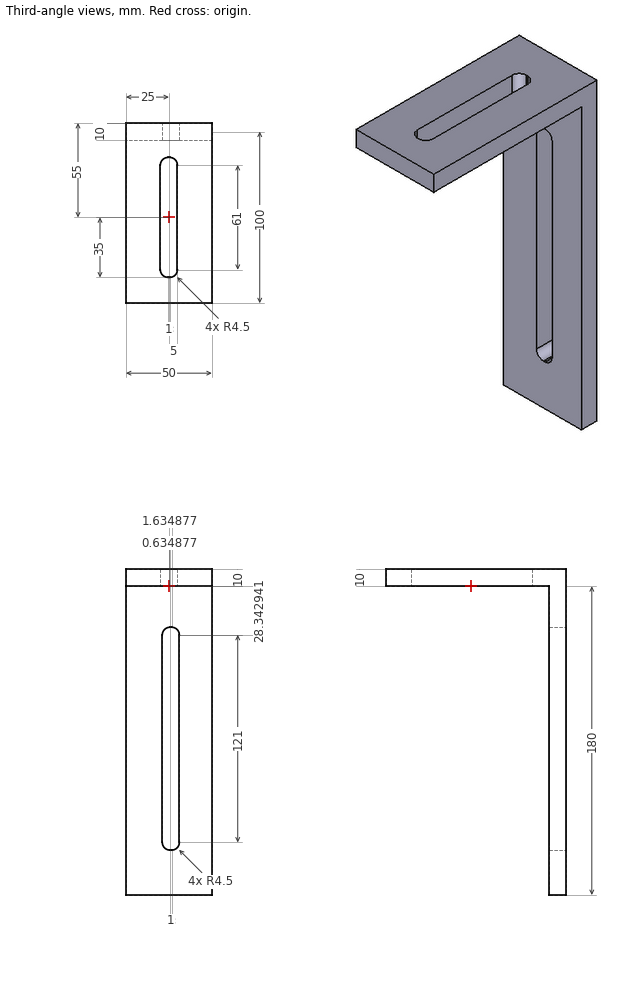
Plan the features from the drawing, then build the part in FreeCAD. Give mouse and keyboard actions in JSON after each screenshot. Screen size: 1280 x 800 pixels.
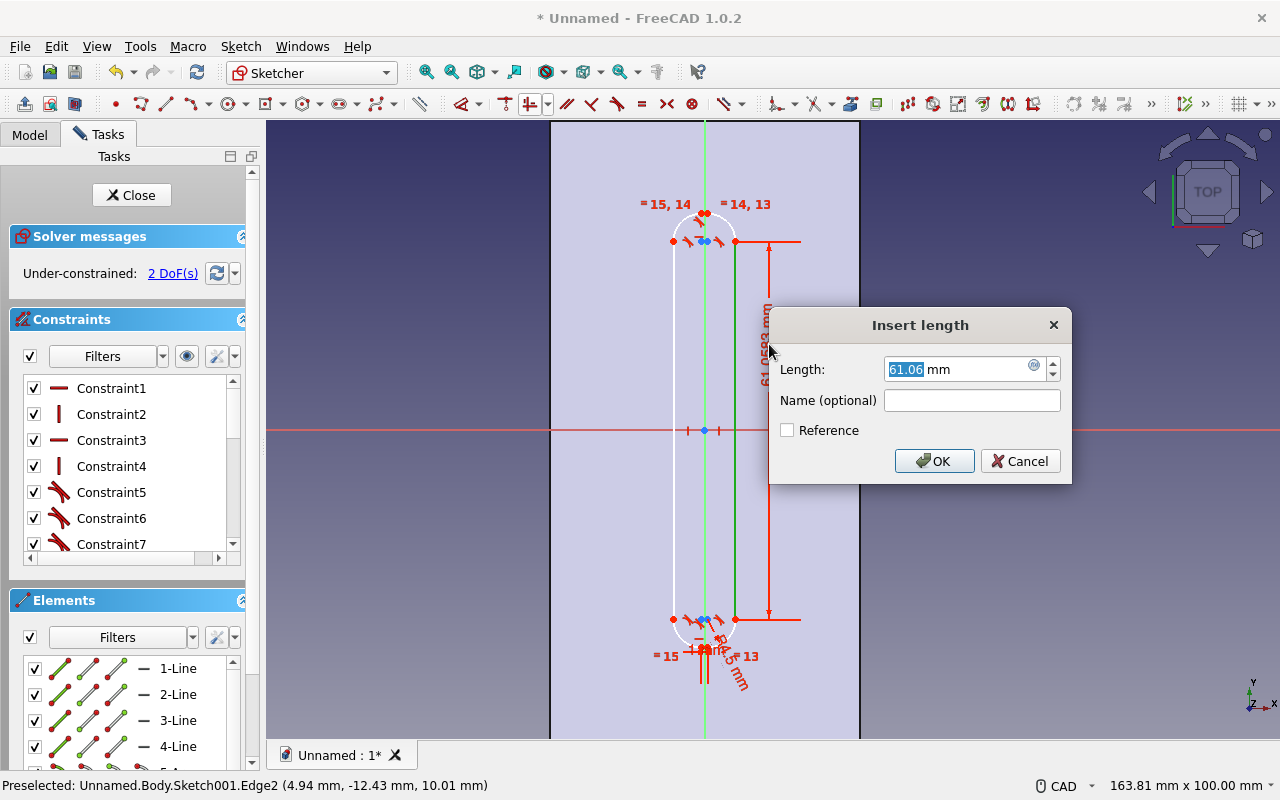
{"action": "type", "text": "61"}
{"action": "key", "text": "Return"}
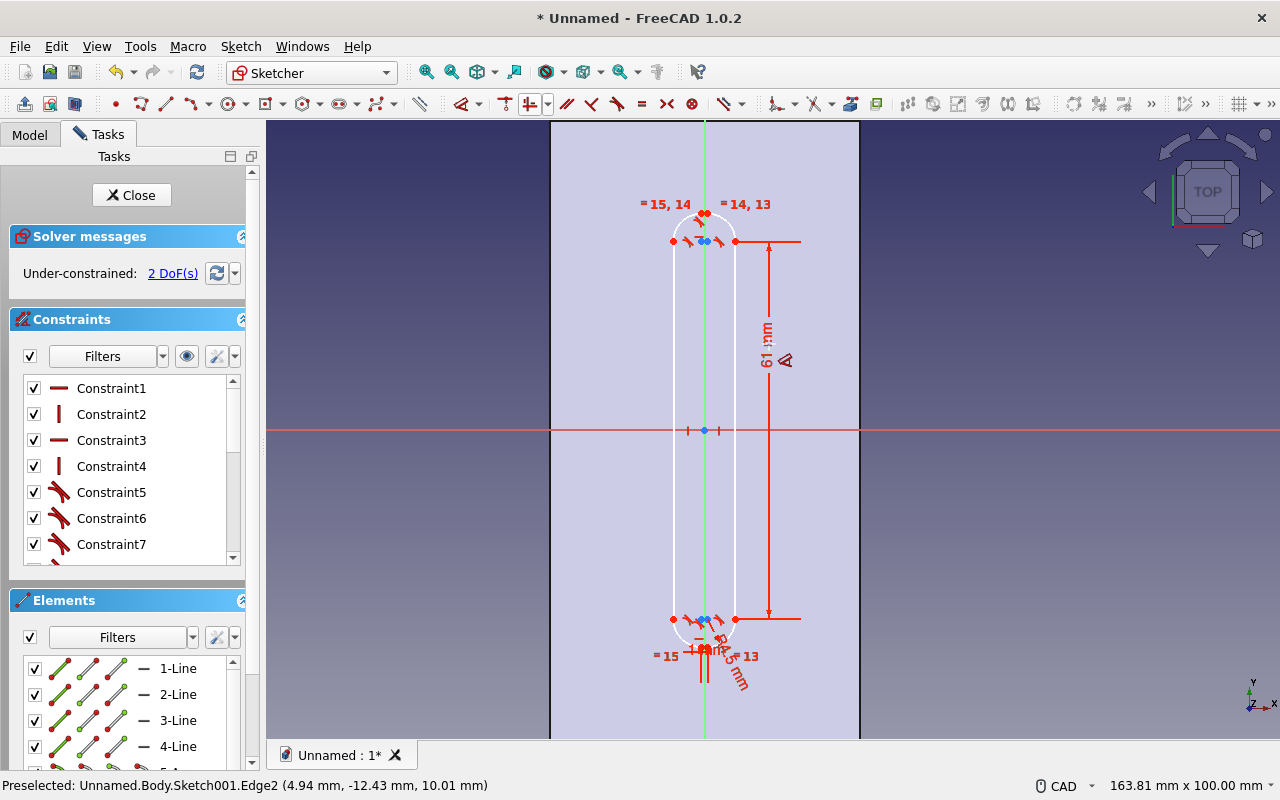
{"action": "scroll", "coordinate": [735, 619], "scroll_direction": "up", "scroll_amount": 2}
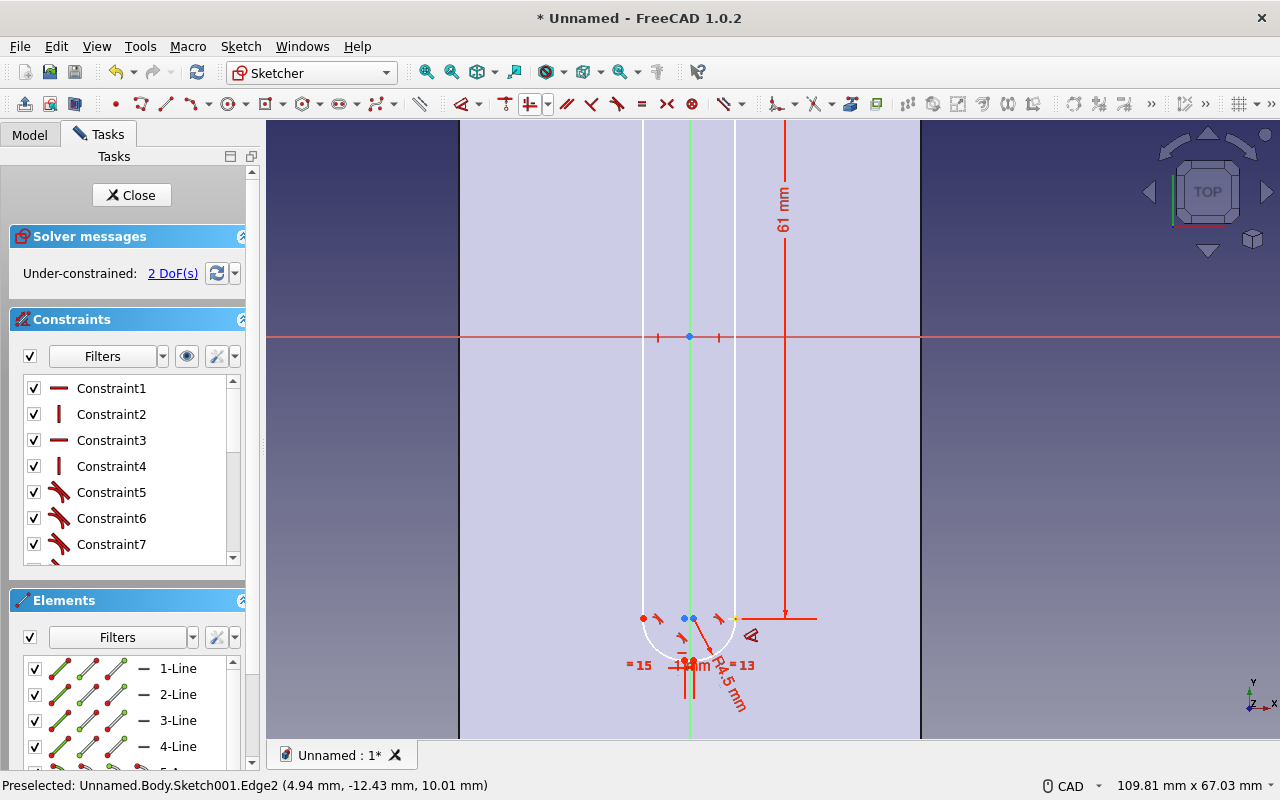
{"action": "left_click", "coordinate": [735, 619]}
{"action": "left_click", "coordinate": [713, 303]}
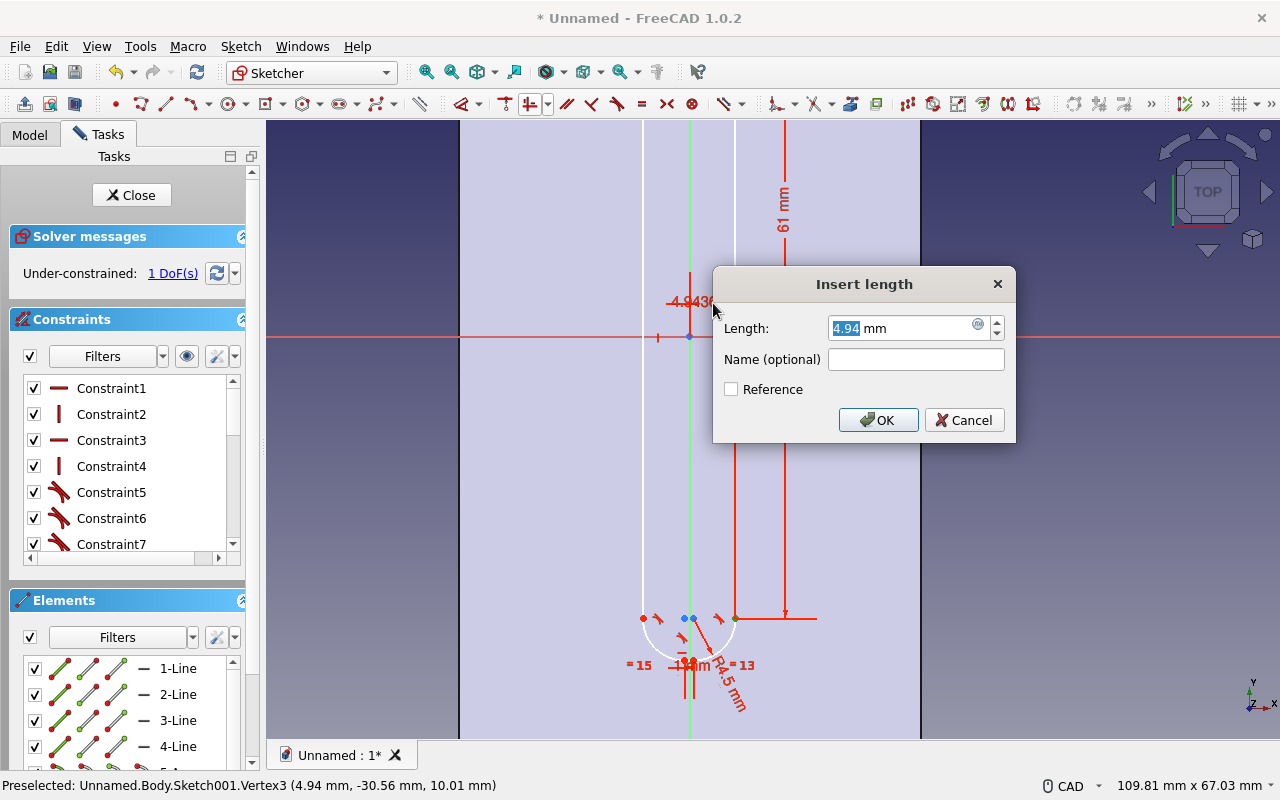
{"action": "type", "text": "5"}
{"action": "key", "text": "Return"}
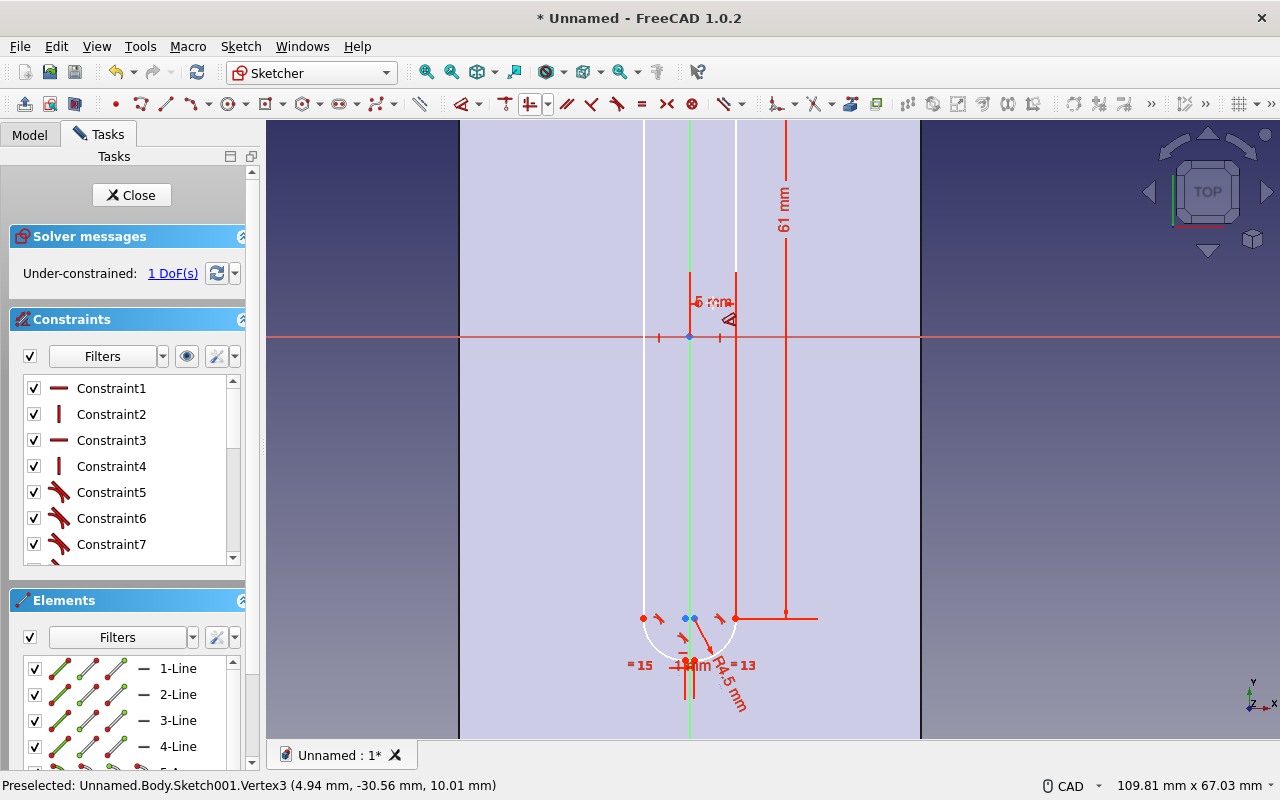
{"action": "scroll", "coordinate": [685, 661], "scroll_direction": "up", "scroll_amount": 2}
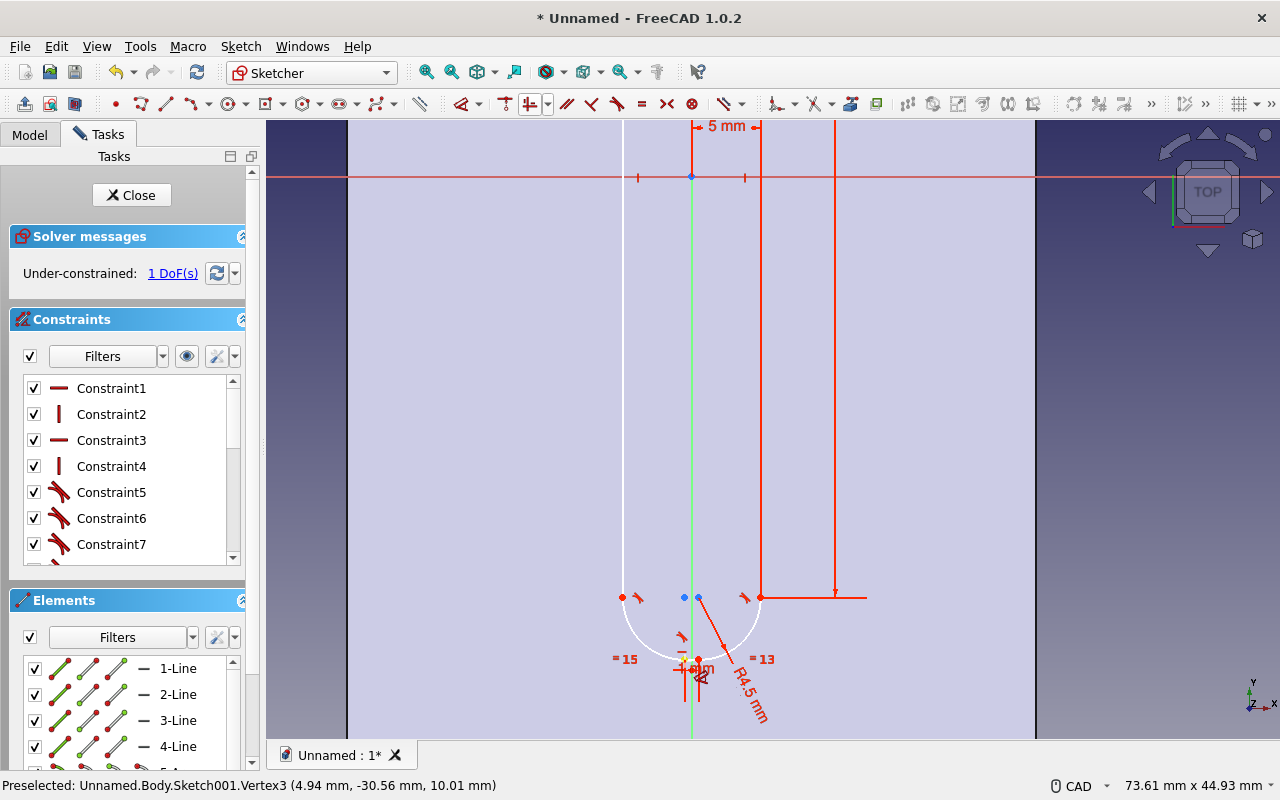
{"action": "left_click", "coordinate": [685, 660]}
{"action": "left_click", "coordinate": [651, 418]}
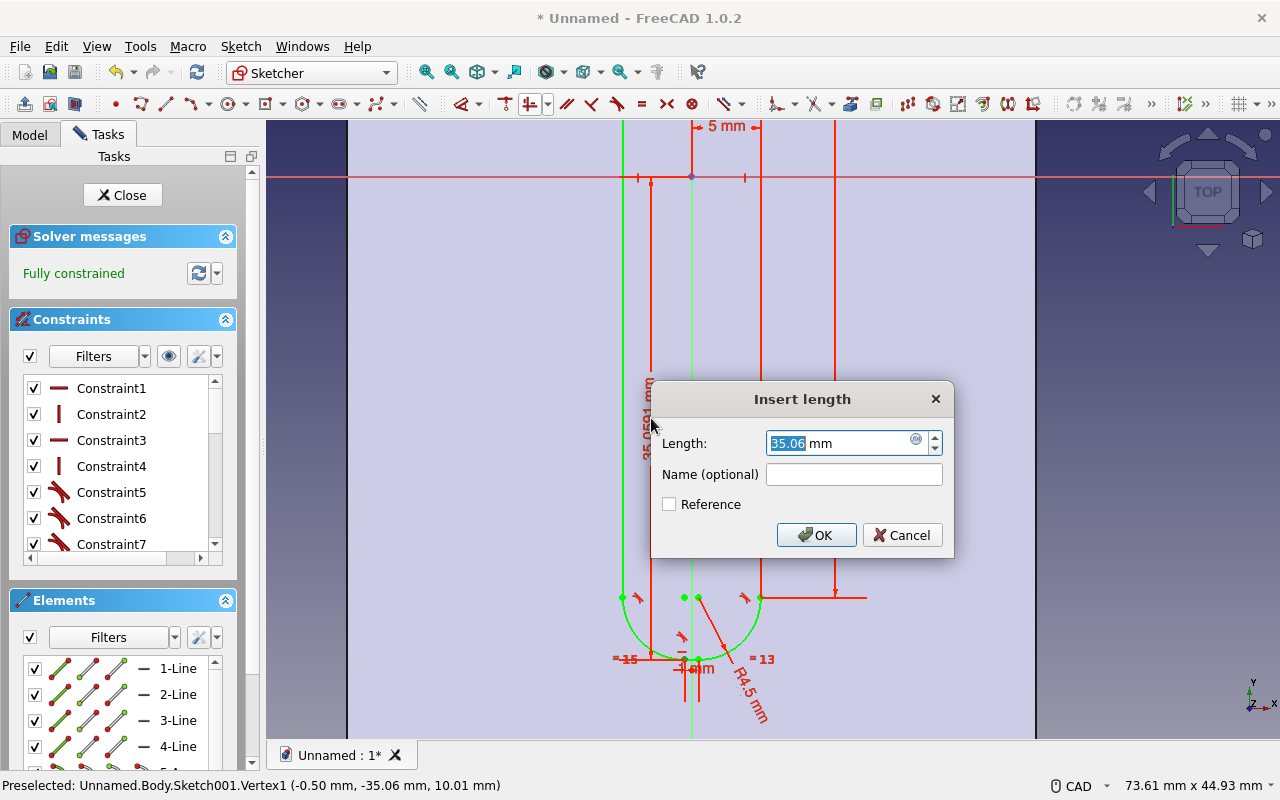
{"action": "type", "text": "35"}
{"action": "key", "text": "Return"}
{"action": "key", "text": "Escape"}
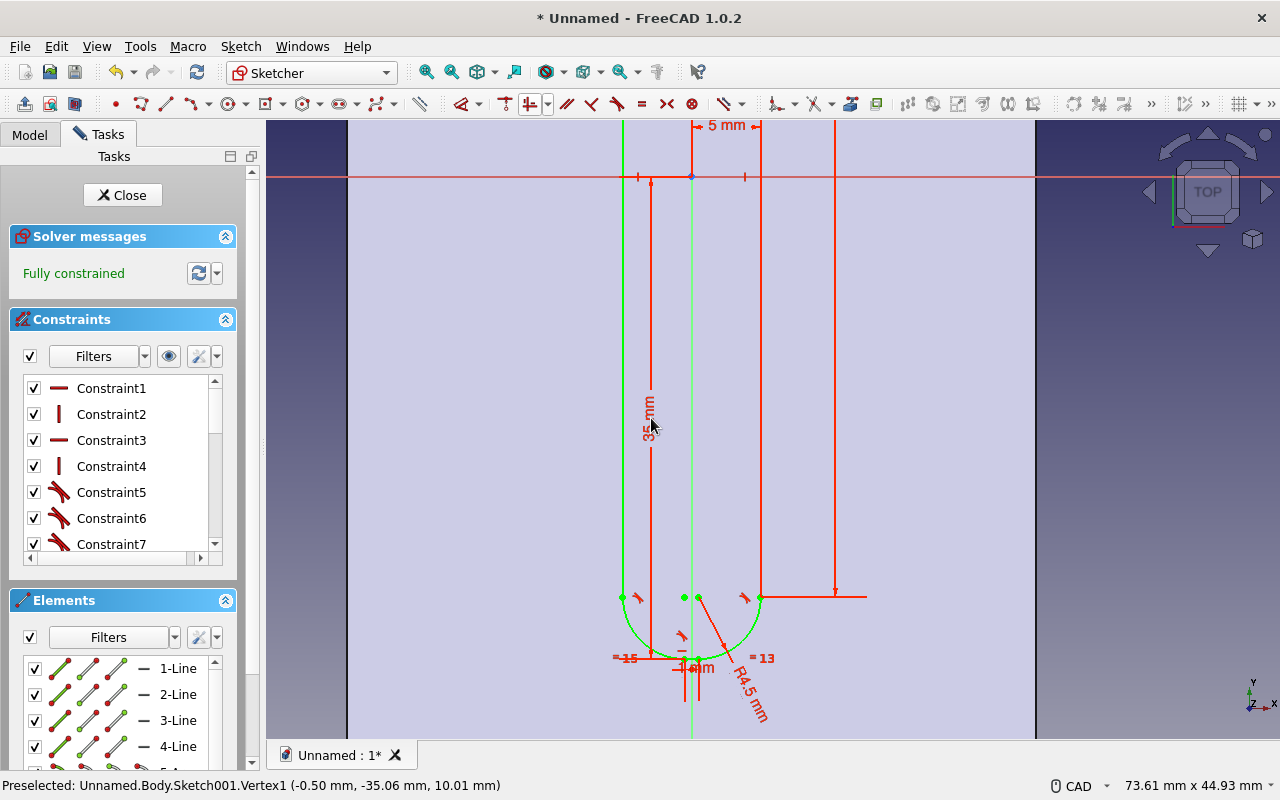
{"action": "left_click", "coordinate": [123, 195]}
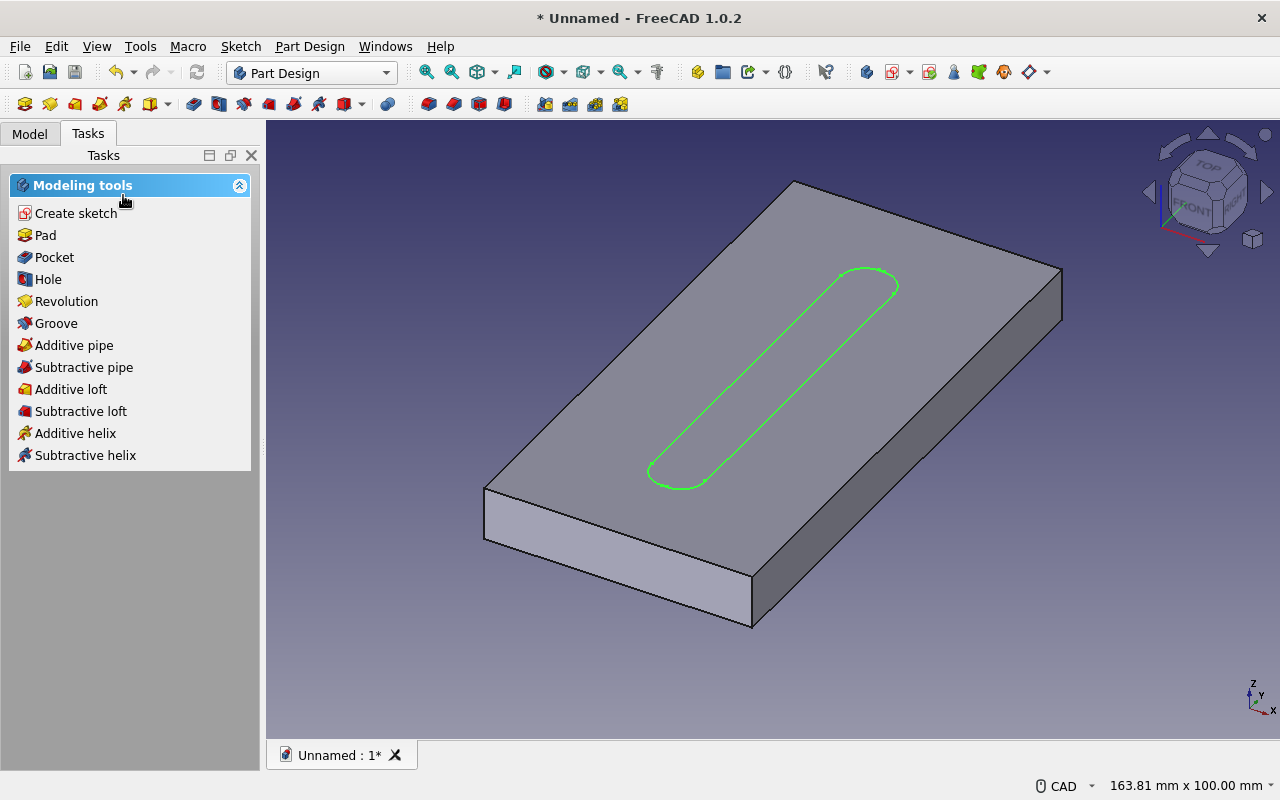
{"action": "left_click", "coordinate": [194, 104]}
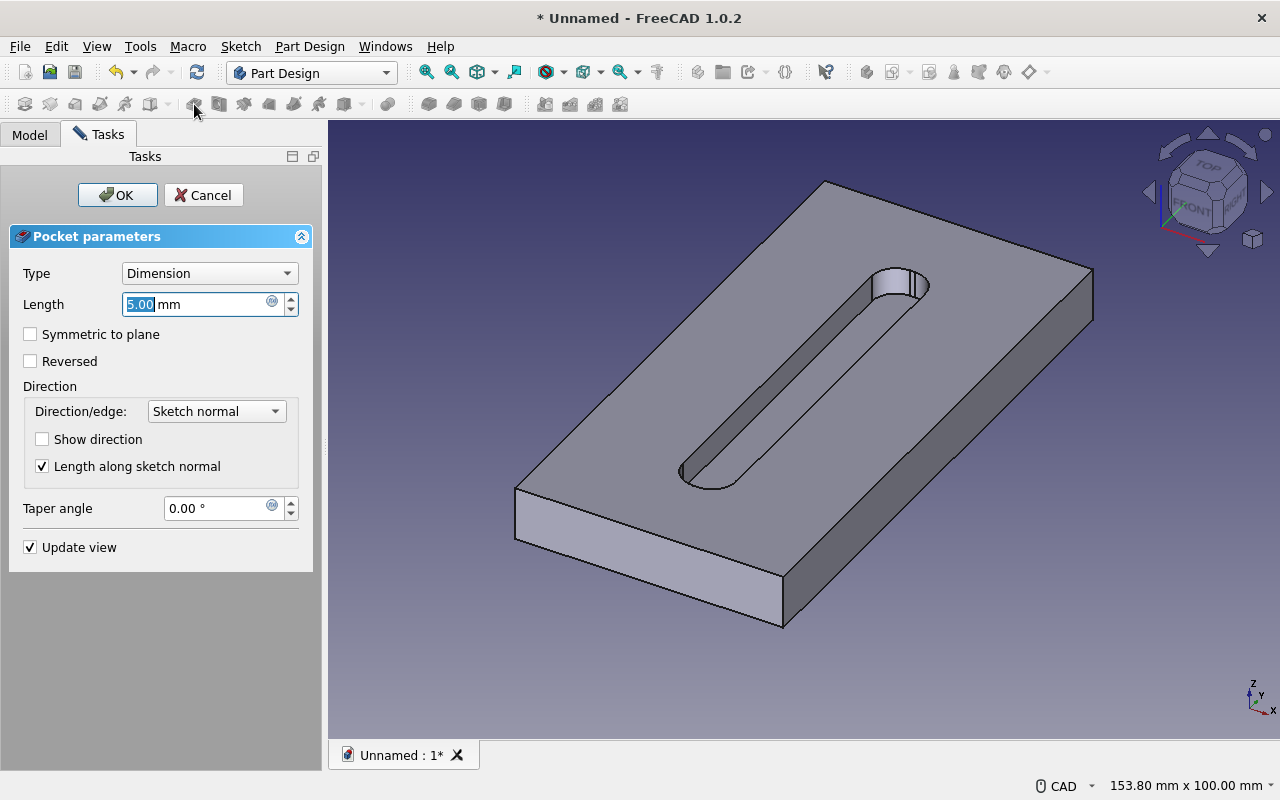
{"action": "type", "text": "10"}
{"action": "key", "text": "Tab"}